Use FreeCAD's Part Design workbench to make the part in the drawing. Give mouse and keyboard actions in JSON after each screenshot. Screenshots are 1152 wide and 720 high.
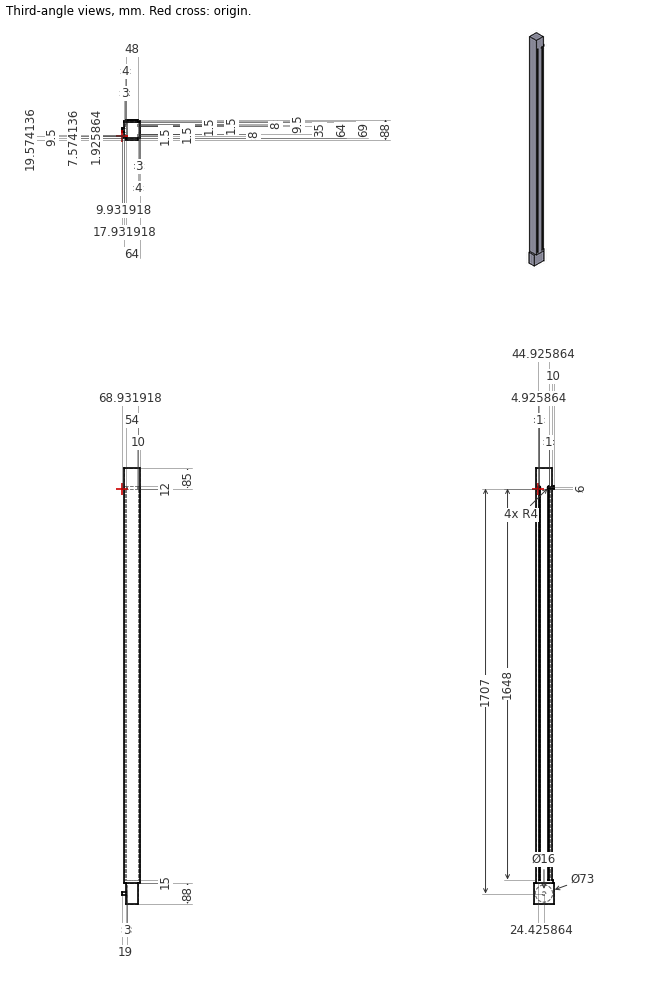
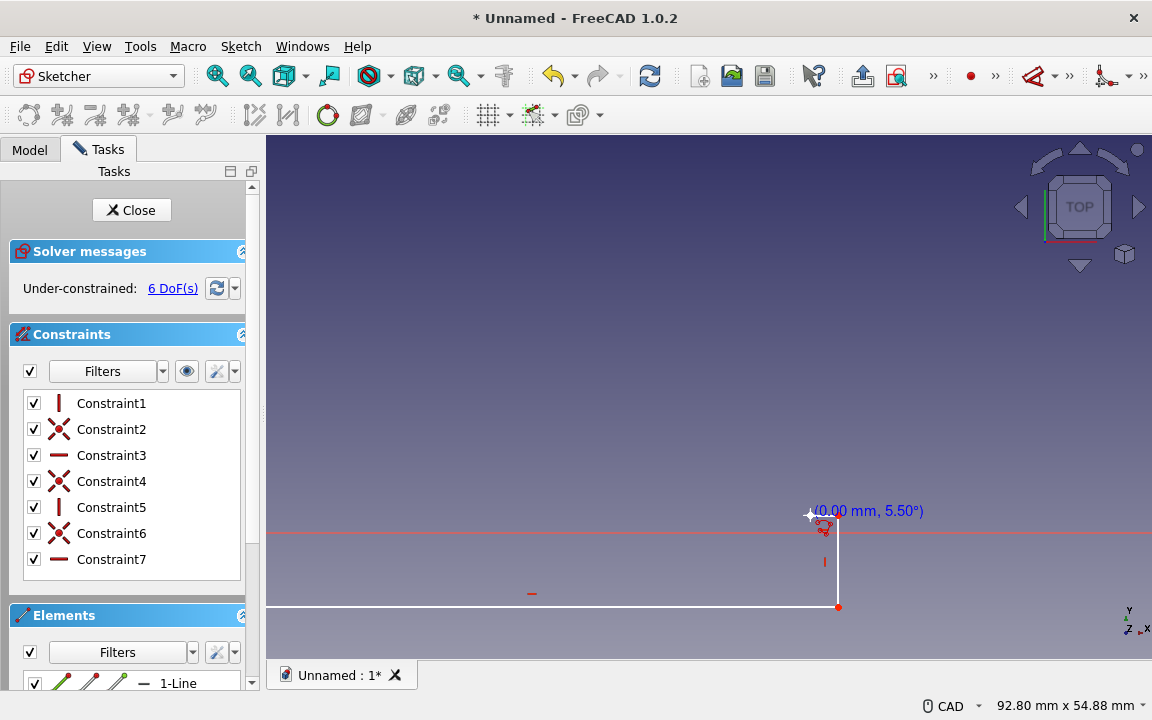
{"action": "scroll", "coordinate": [810, 529], "scroll_direction": "up", "scroll_amount": 7}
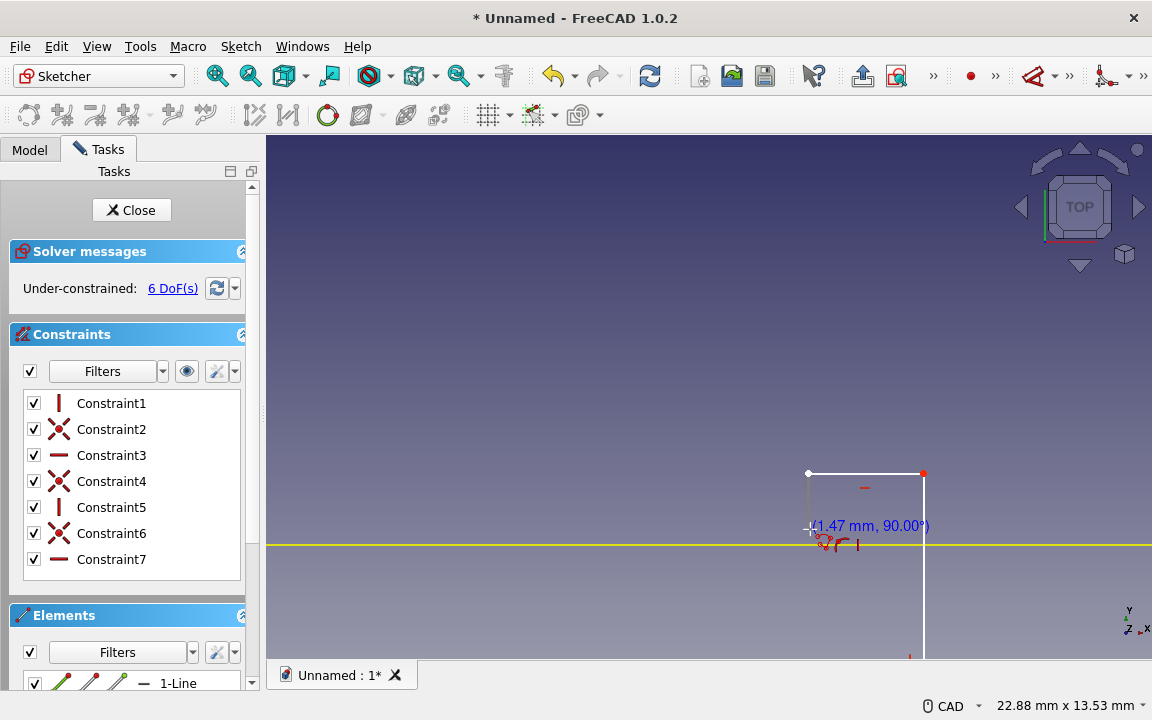
{"action": "left_click", "coordinate": [808, 528]}
{"action": "left_click", "coordinate": [654, 528]}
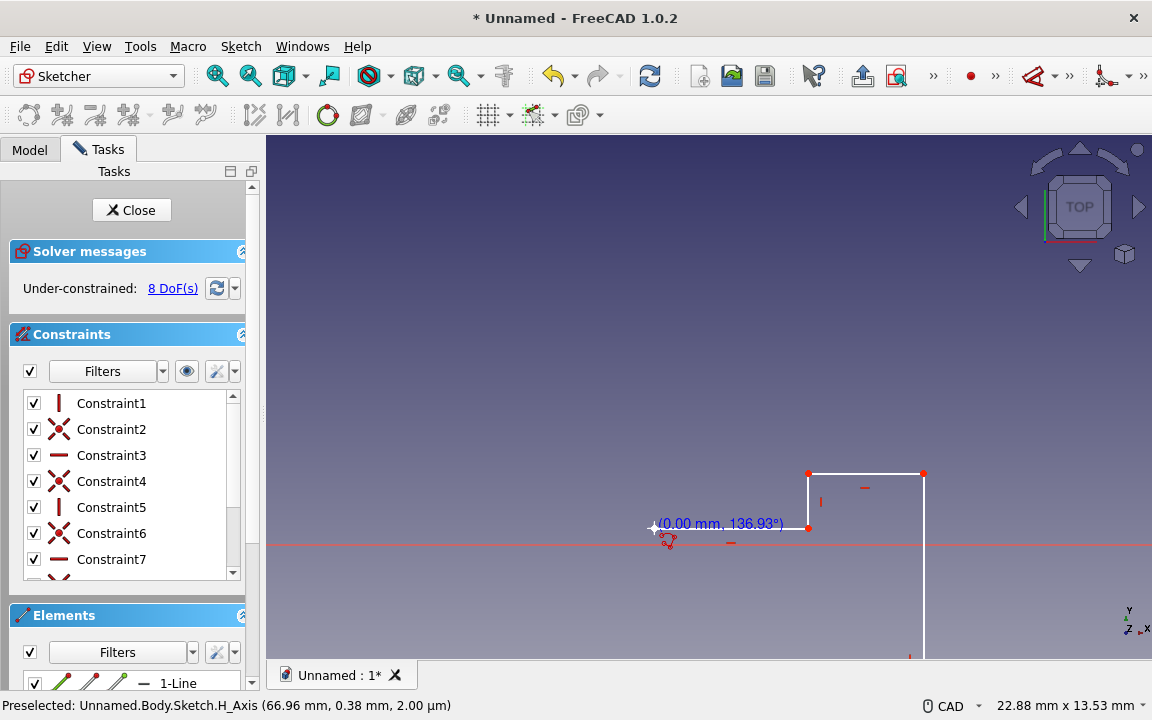
{"action": "scroll", "coordinate": [820, 522], "scroll_direction": "down", "scroll_amount": 10}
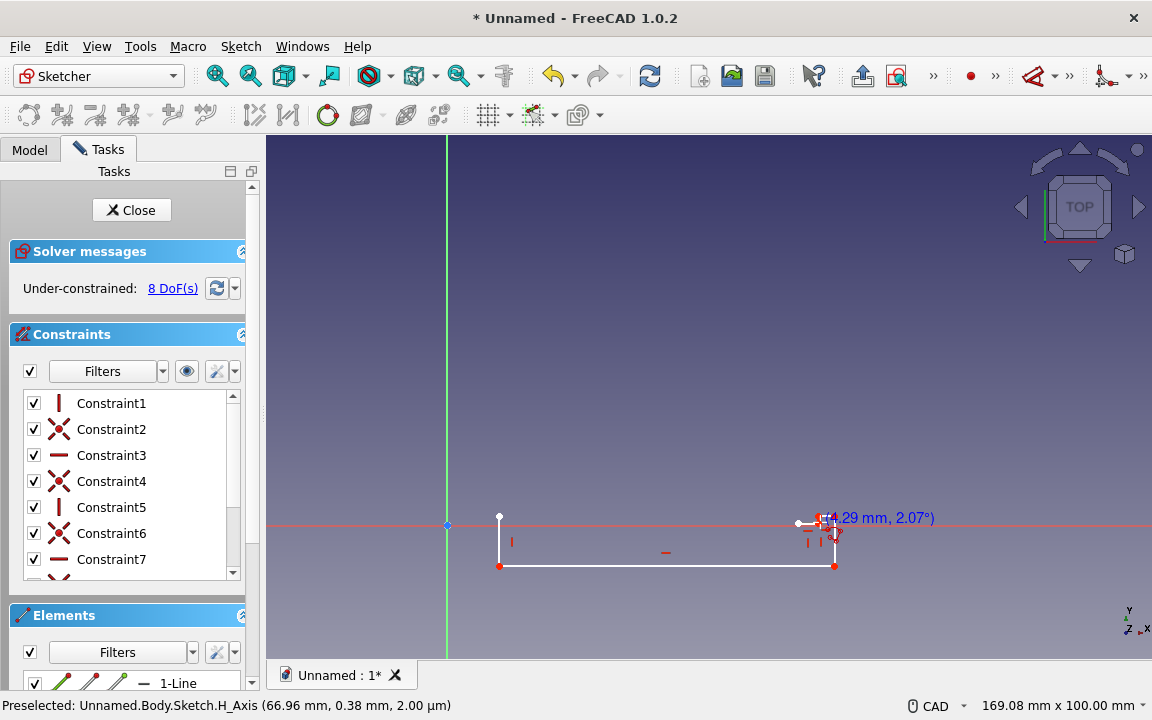
{"action": "left_click", "coordinate": [798, 482]}
{"action": "left_click", "coordinate": [819, 482]}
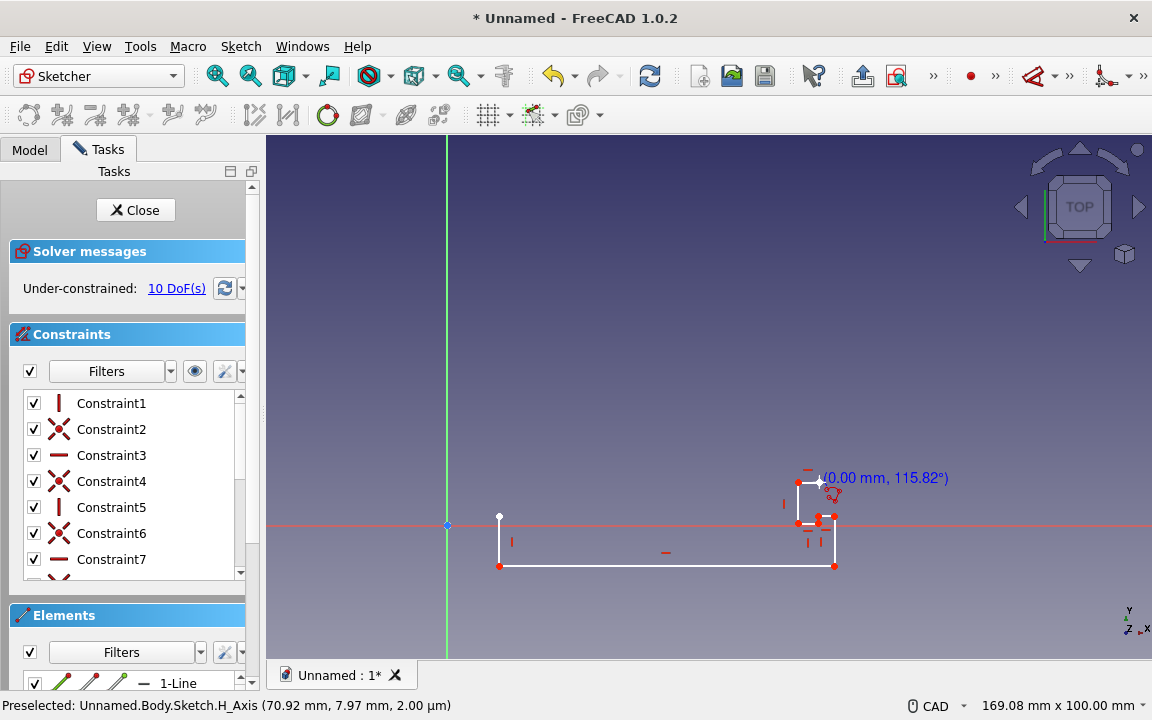
{"action": "scroll", "coordinate": [819, 489], "scroll_direction": "up", "scroll_amount": 4}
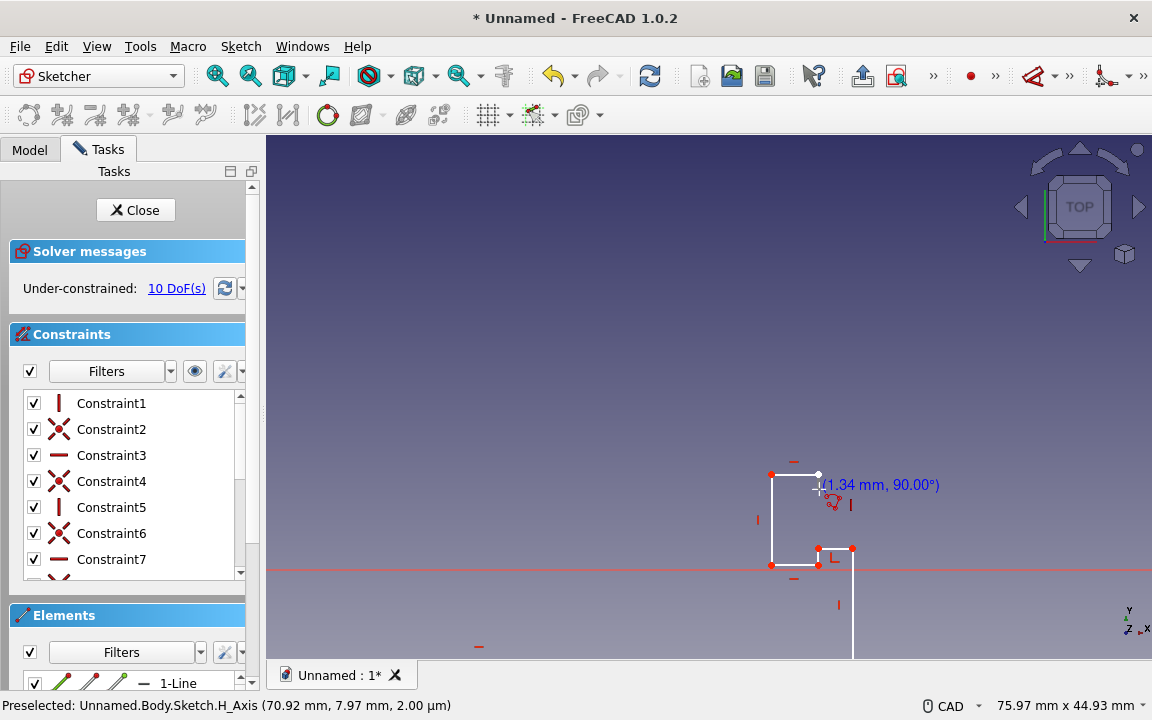
{"action": "left_click", "coordinate": [818, 489]}
{"action": "left_click", "coordinate": [853, 489]}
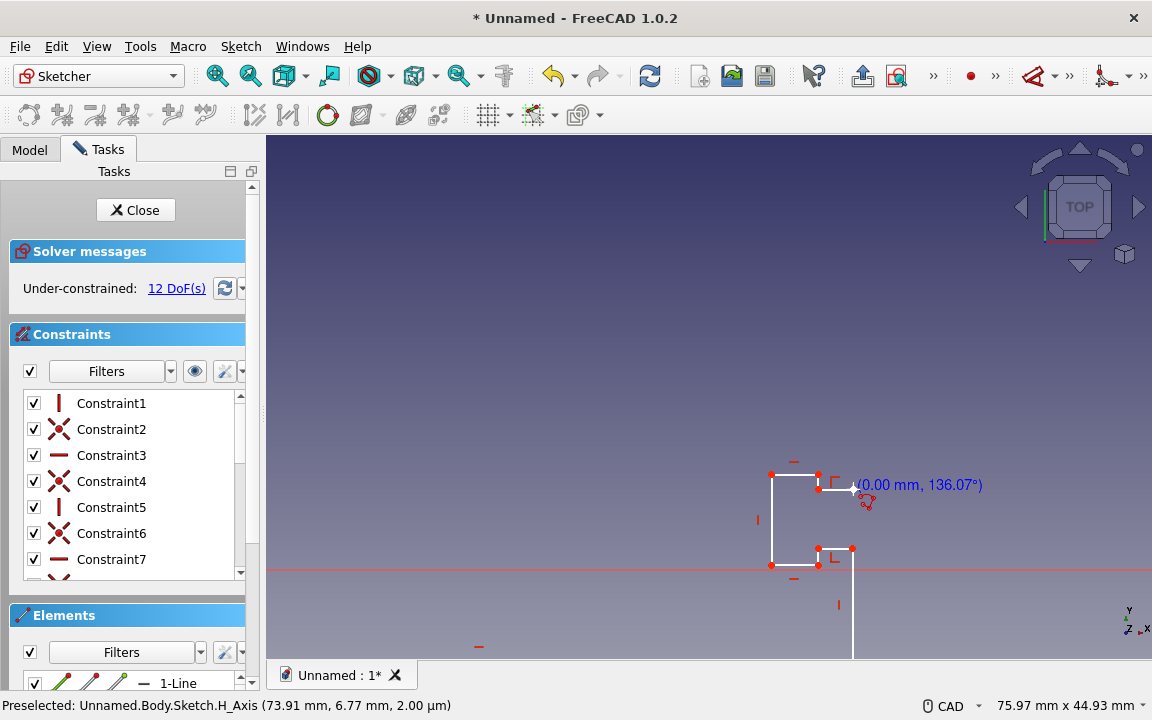
{"action": "scroll", "coordinate": [819, 488], "scroll_direction": "down", "scroll_amount": 4}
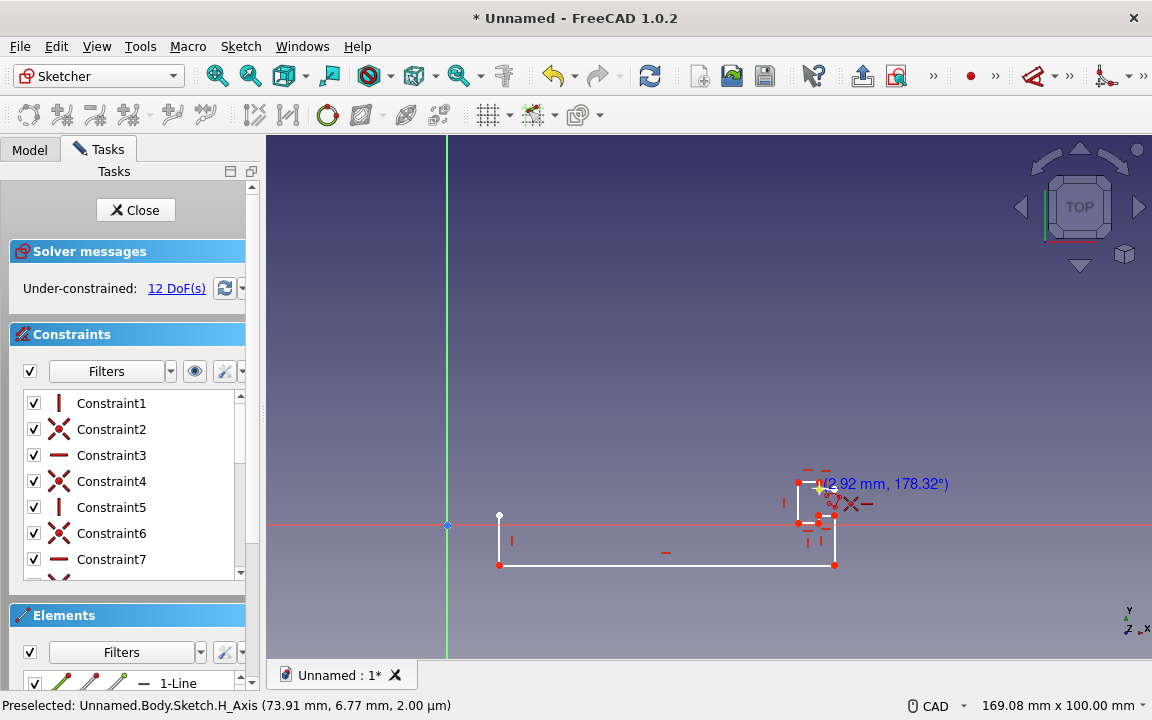
{"action": "left_click", "coordinate": [835, 305]}
{"action": "left_click", "coordinate": [819, 305]}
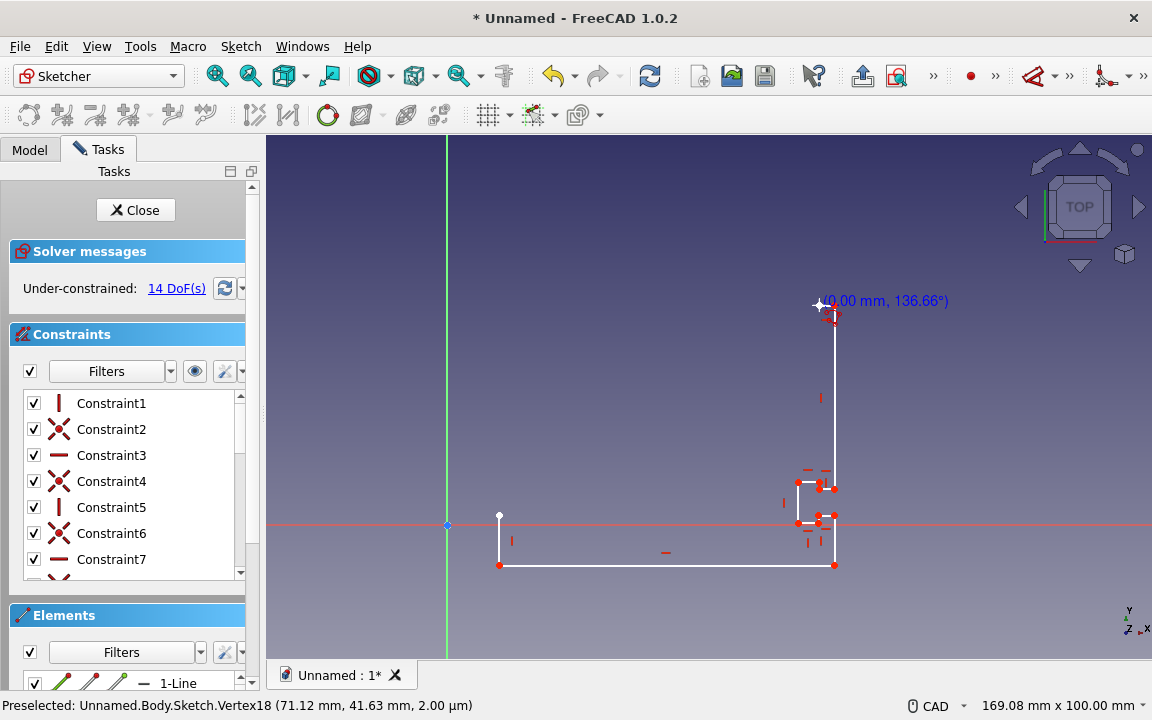
{"action": "scroll", "coordinate": [819, 313], "scroll_direction": "up", "scroll_amount": 4}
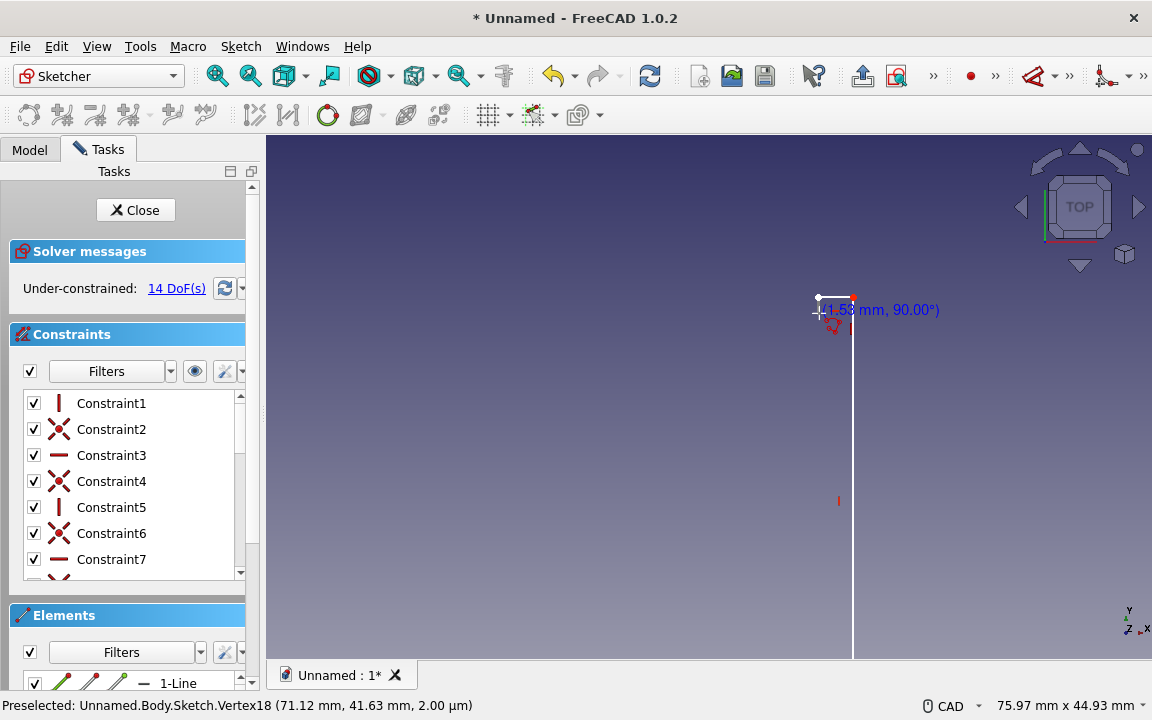
{"action": "left_click", "coordinate": [818, 313]}
{"action": "left_click", "coordinate": [772, 313]}
{"action": "left_click", "coordinate": [772, 220]}
{"action": "left_click", "coordinate": [818, 220]}
{"action": "left_click", "coordinate": [818, 238]}
{"action": "left_click", "coordinate": [853, 238]}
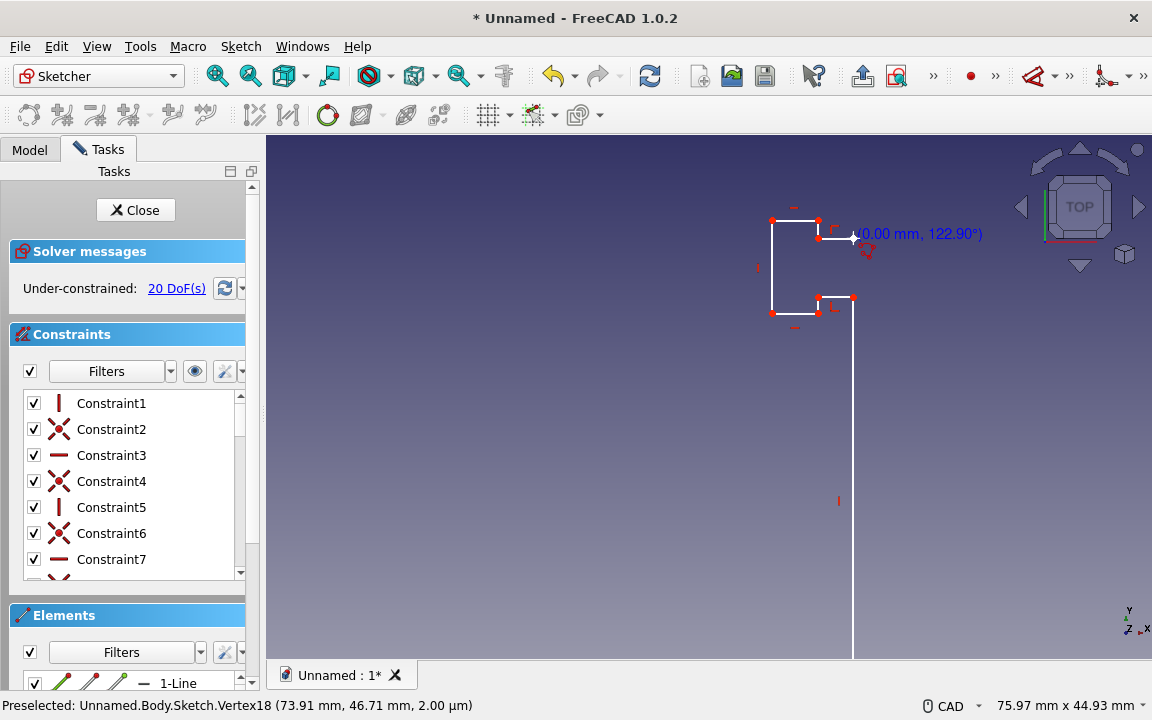
{"action": "scroll", "coordinate": [819, 313], "scroll_direction": "down", "scroll_amount": 4}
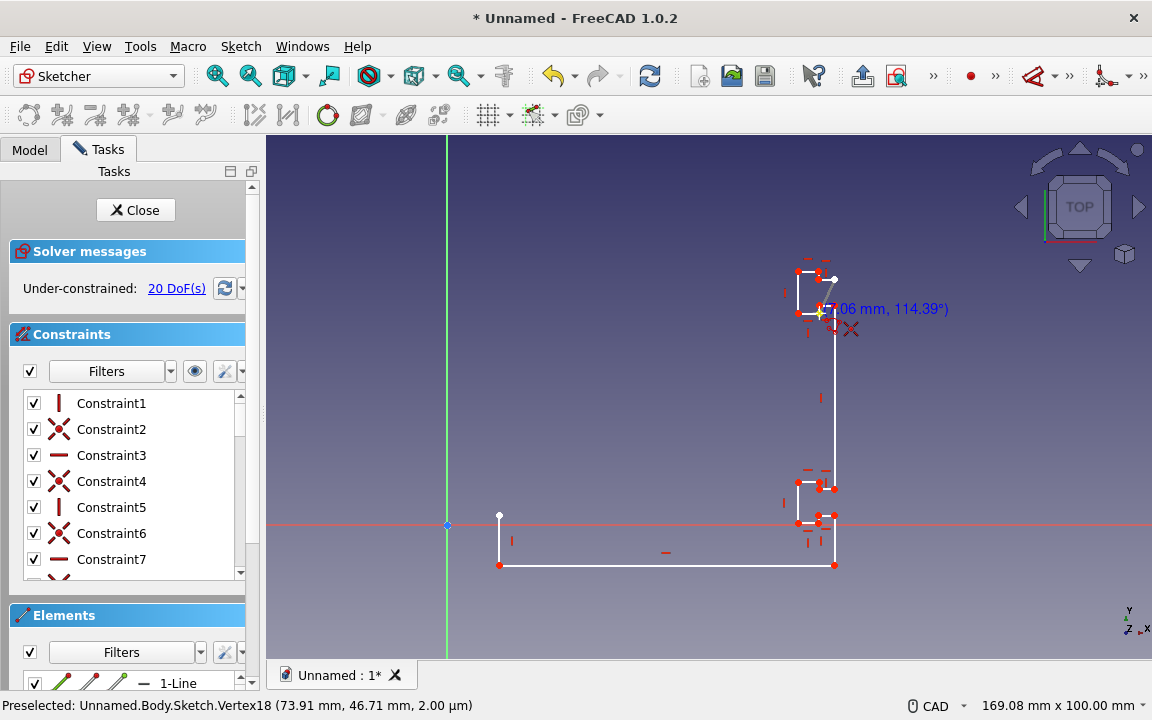
{"action": "left_click", "coordinate": [835, 229]}
{"action": "left_click", "coordinate": [499, 229]}
{"action": "left_click", "coordinate": [499, 279]}
{"action": "left_click", "coordinate": [515, 279]}